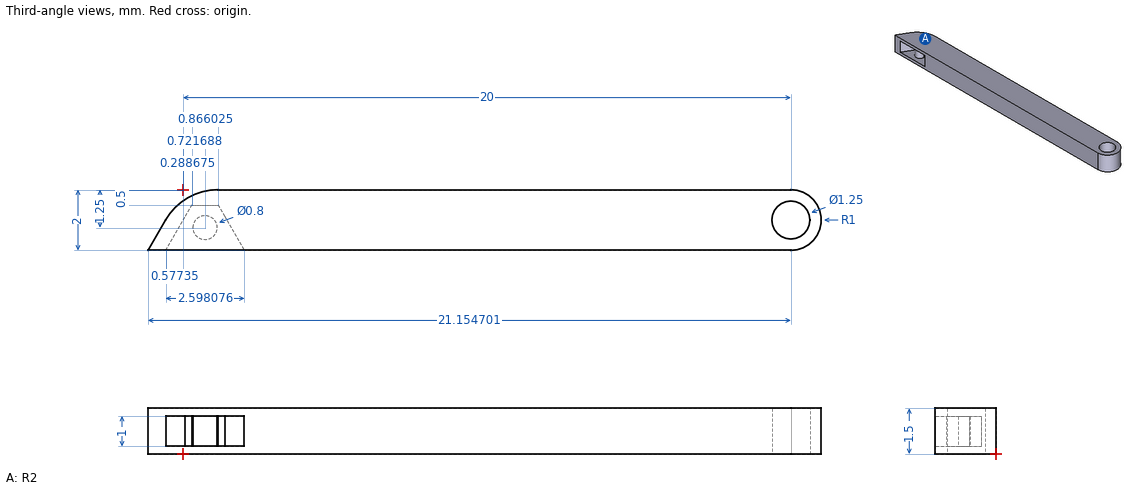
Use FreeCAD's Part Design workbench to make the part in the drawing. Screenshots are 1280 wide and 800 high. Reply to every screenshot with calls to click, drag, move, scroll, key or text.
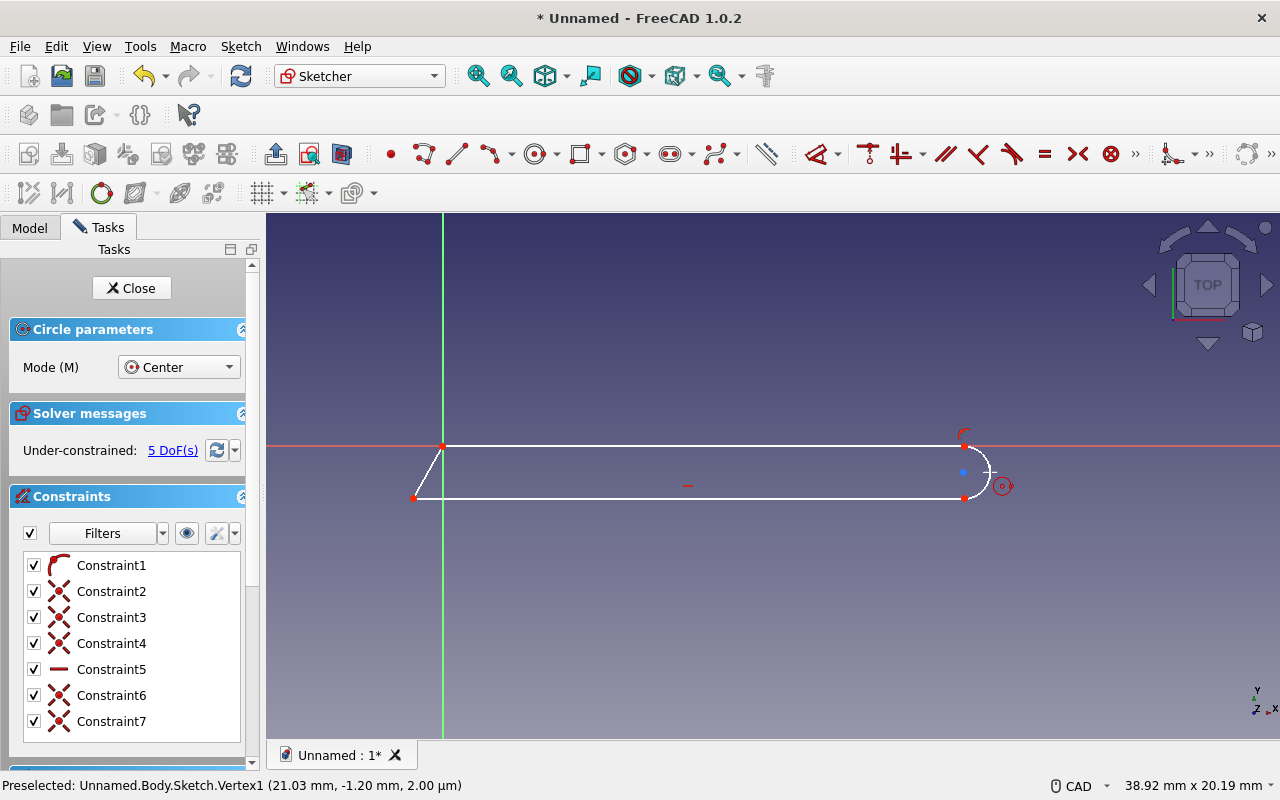
scroll(964, 472, up, 2)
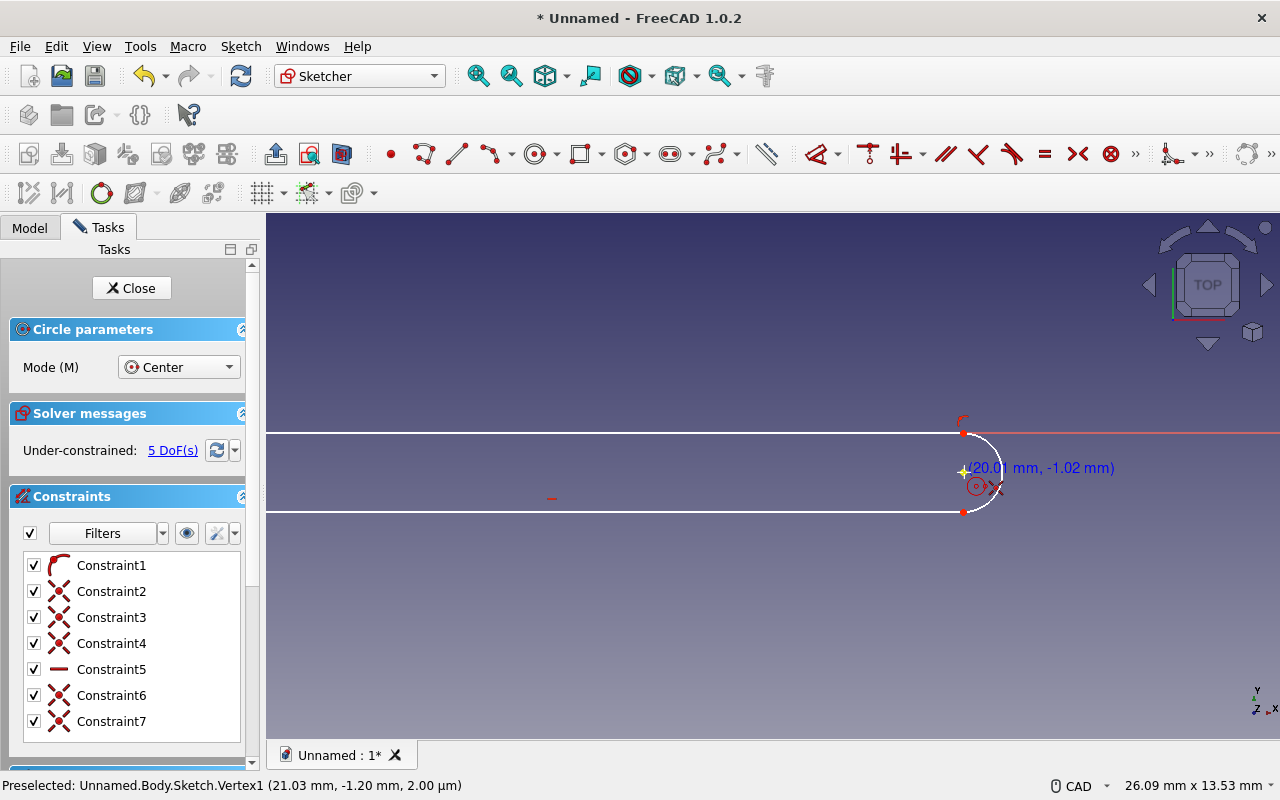
click(963, 472)
move(980, 455)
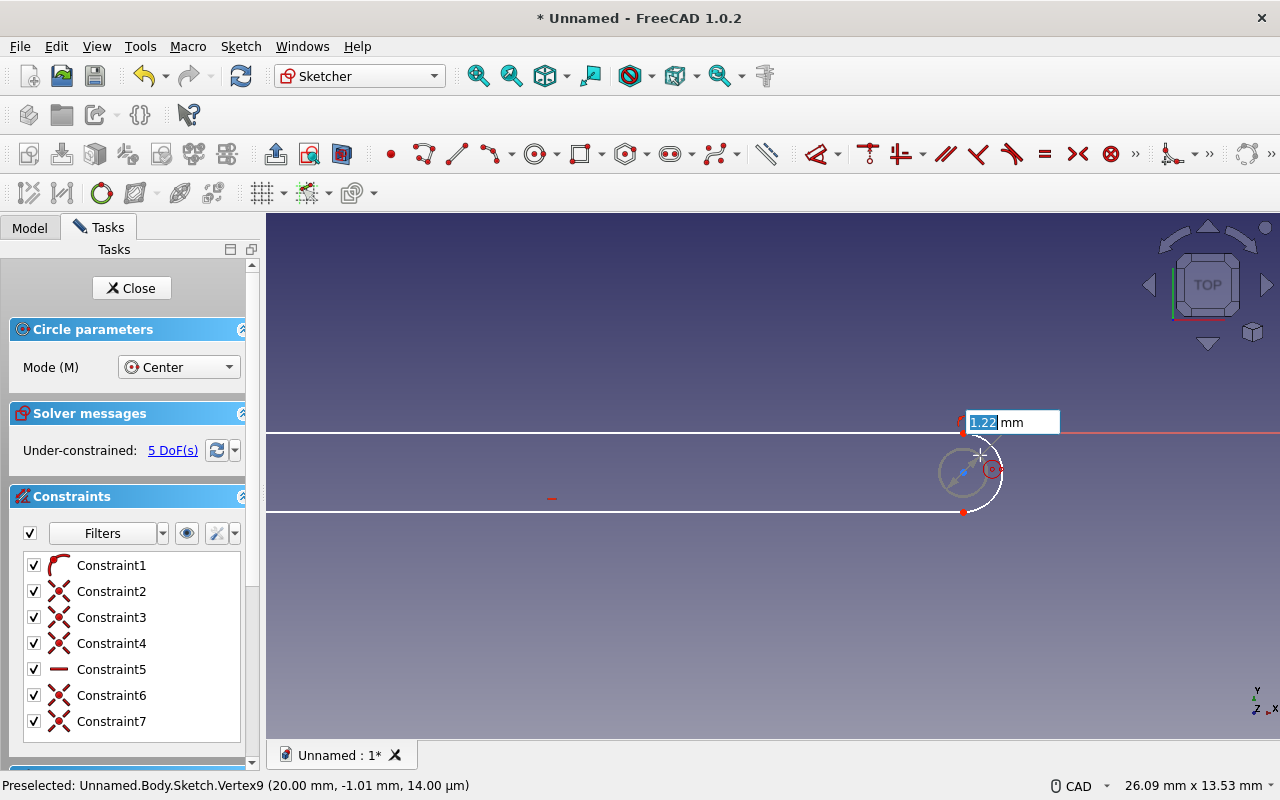
text(1.25)
key(Return)
key(Escape)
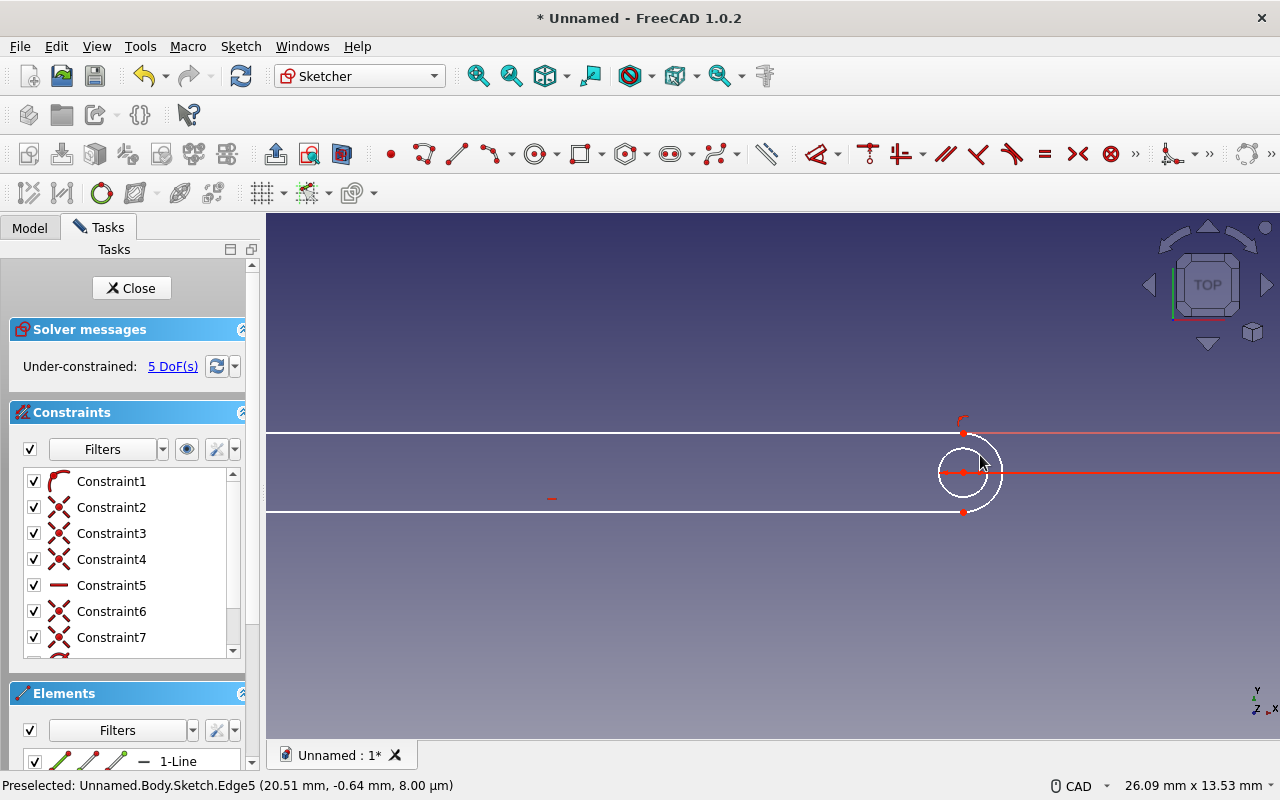
click(730, 433)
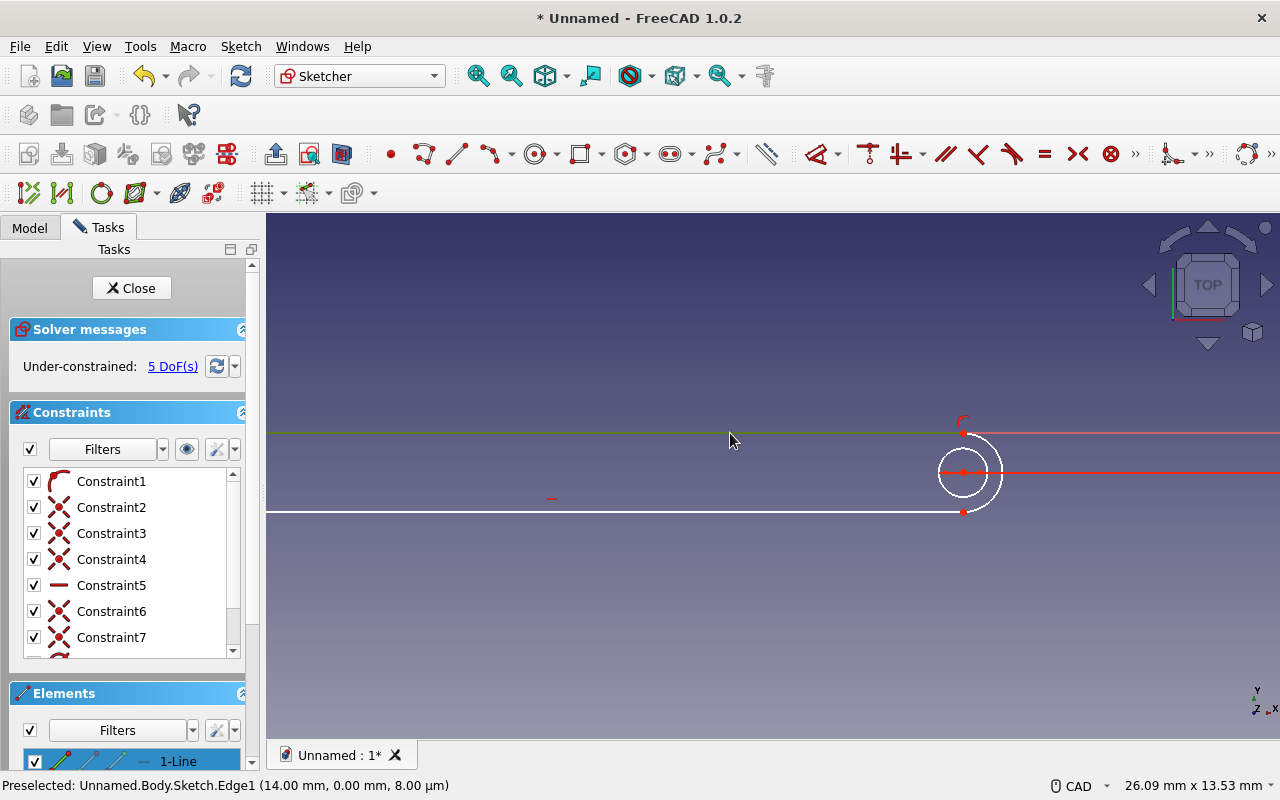
click(995, 496)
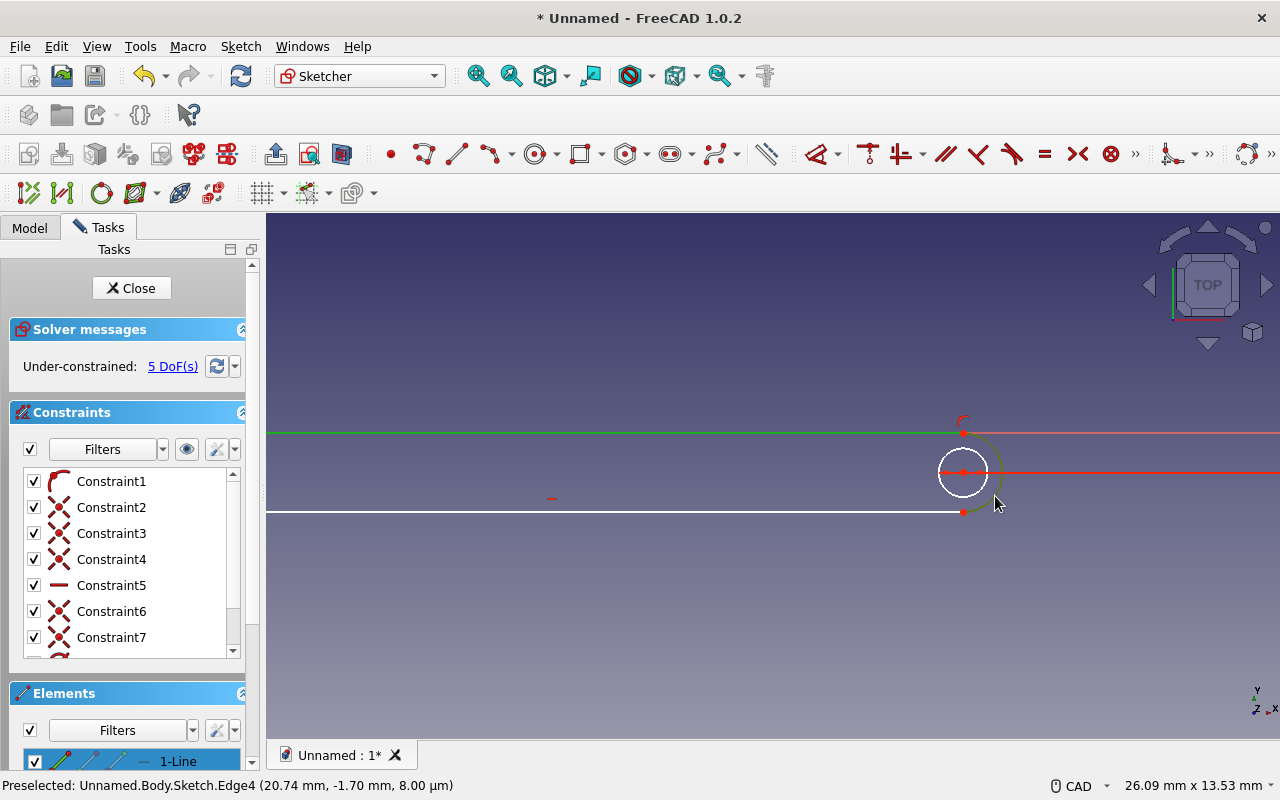
click(1012, 154)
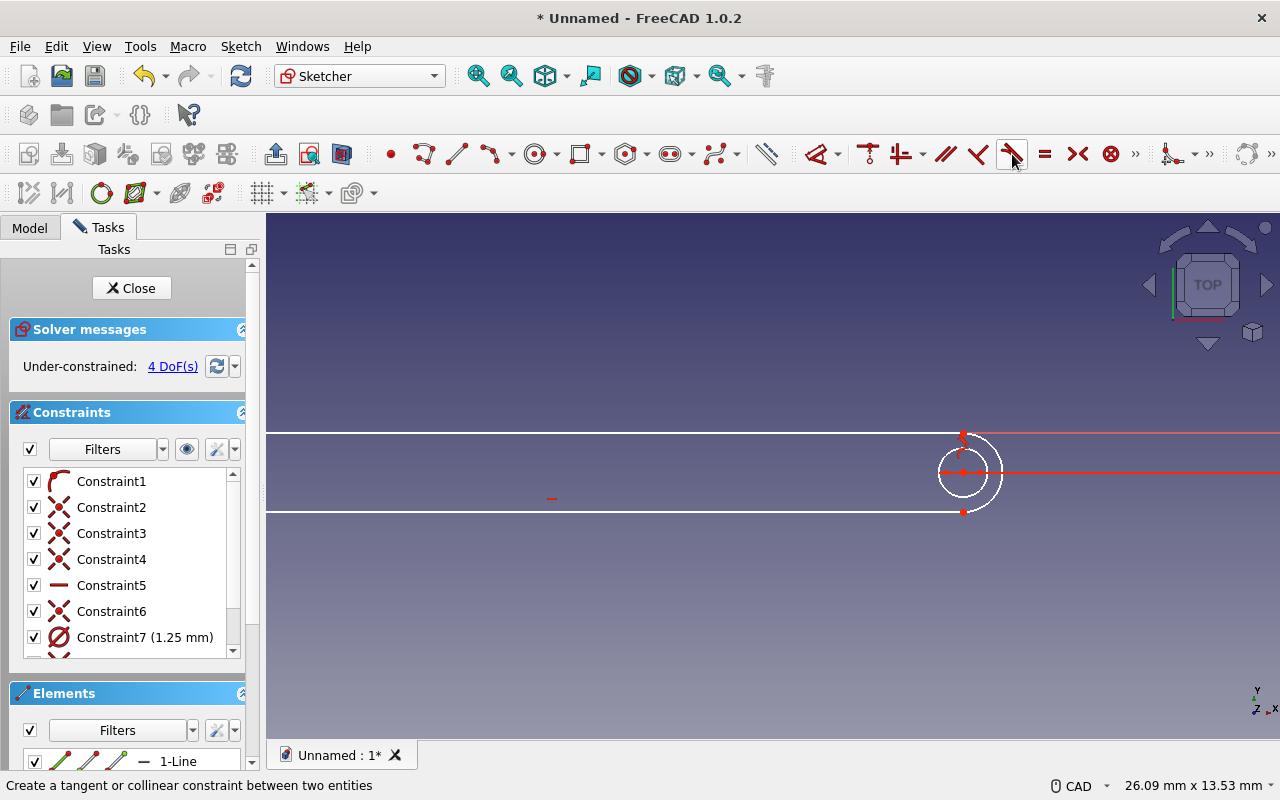
click(388, 512)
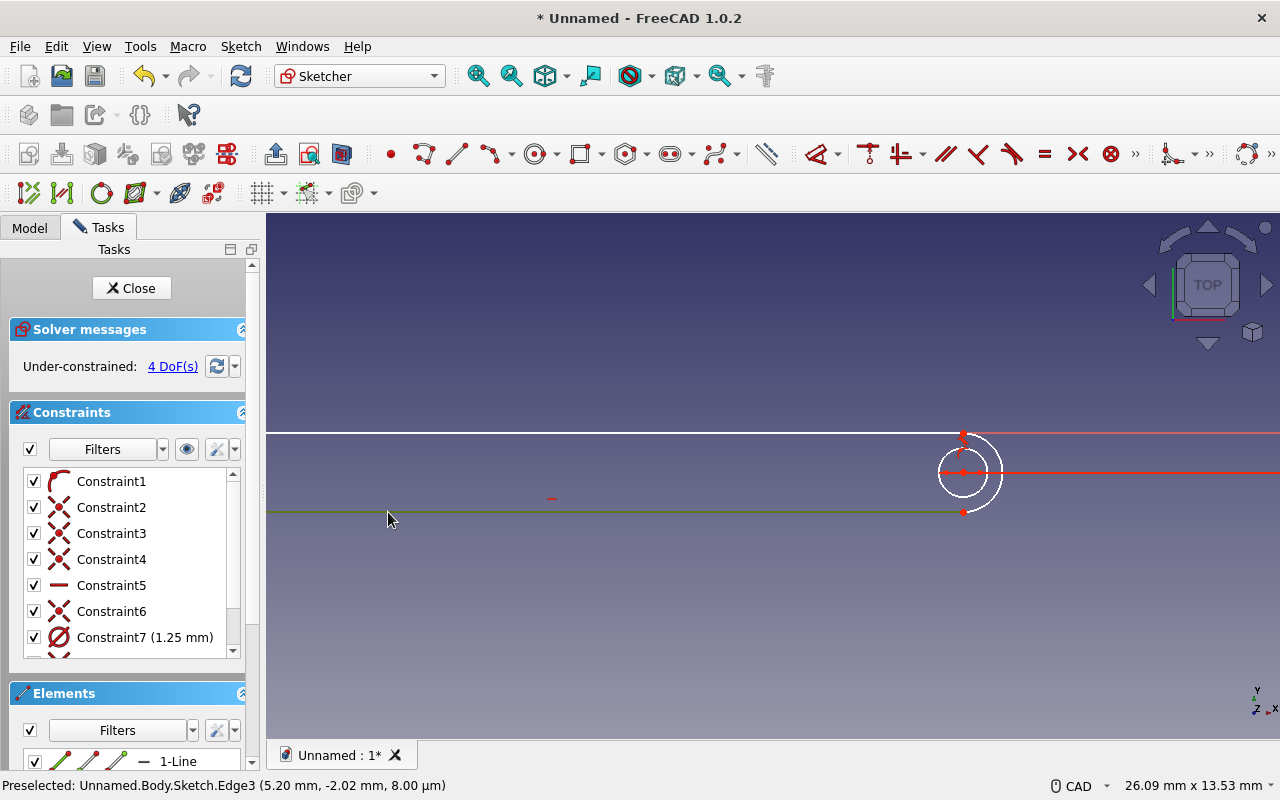
click(995, 496)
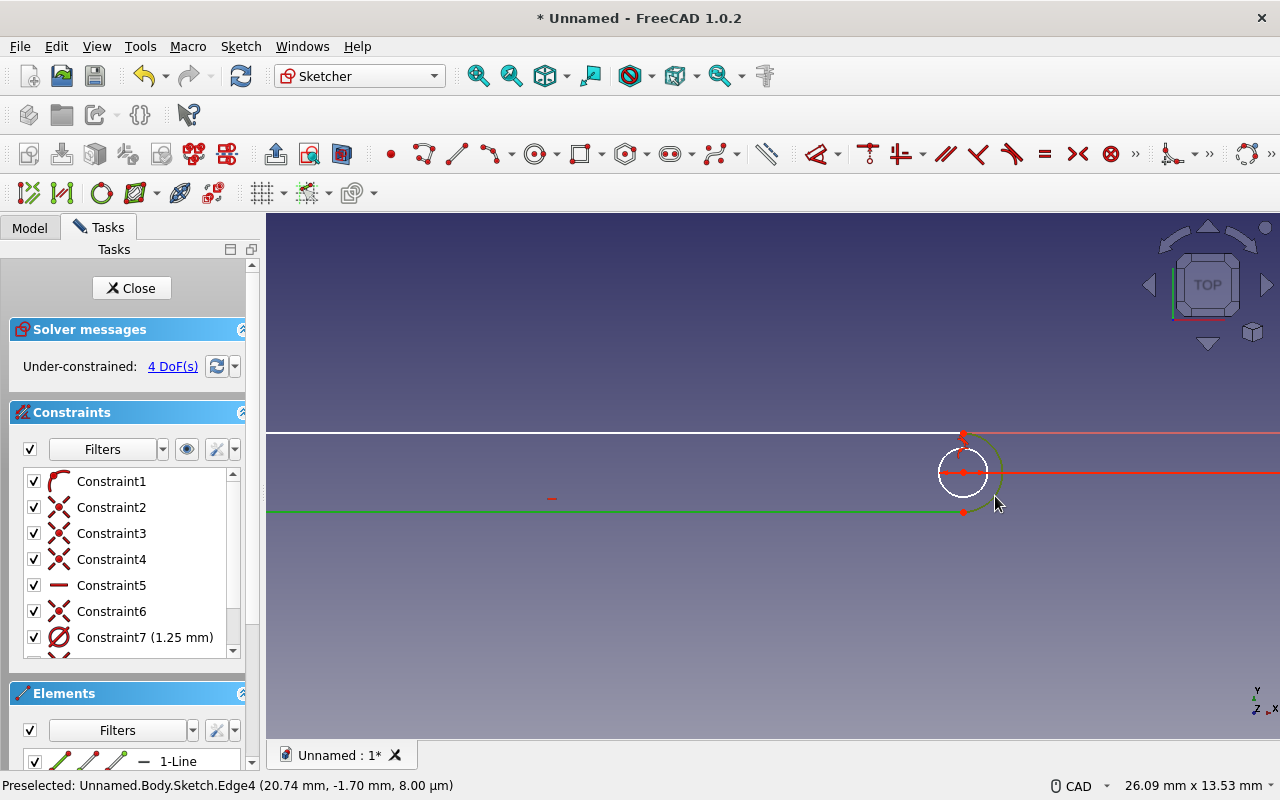
key(t)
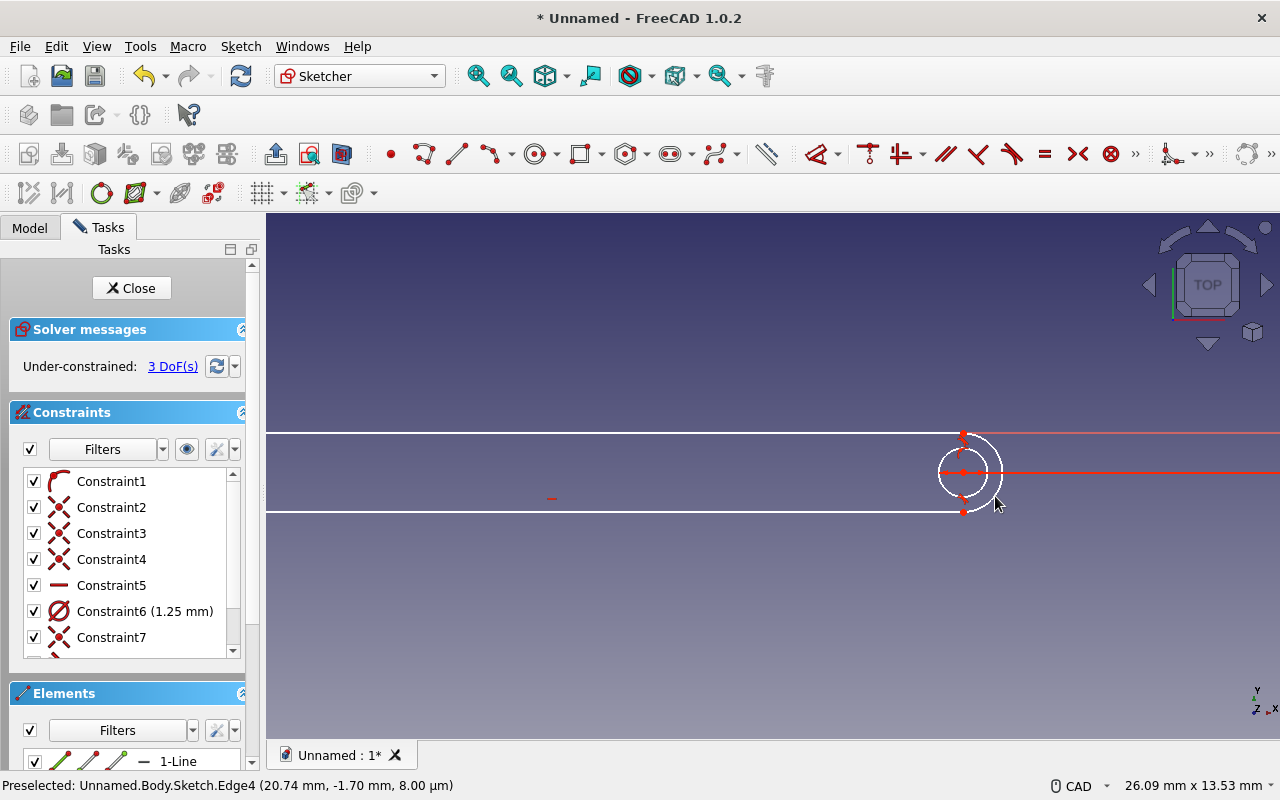
click(816, 154)